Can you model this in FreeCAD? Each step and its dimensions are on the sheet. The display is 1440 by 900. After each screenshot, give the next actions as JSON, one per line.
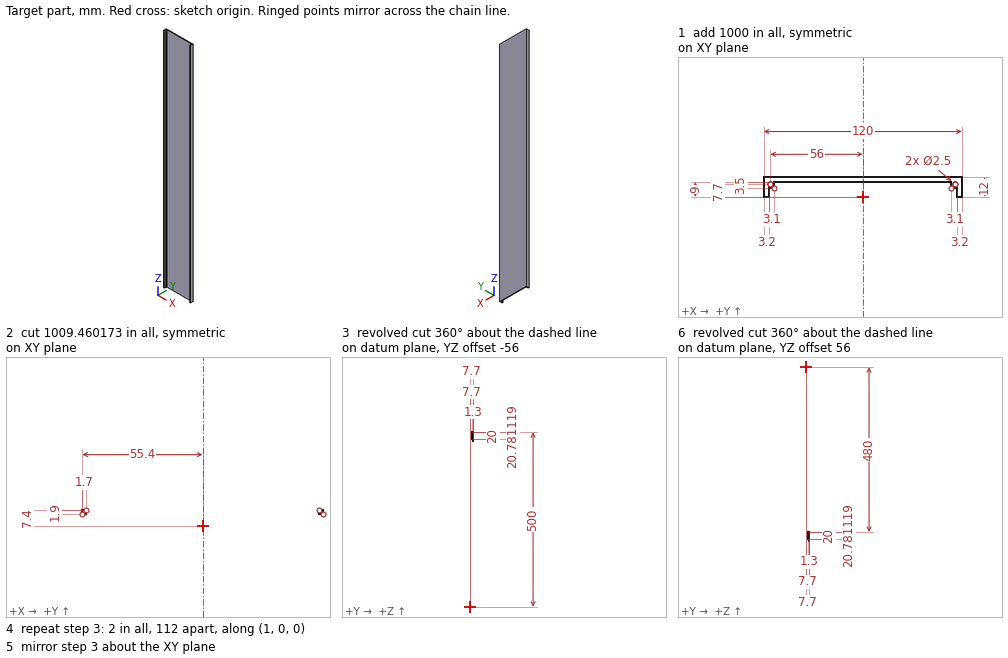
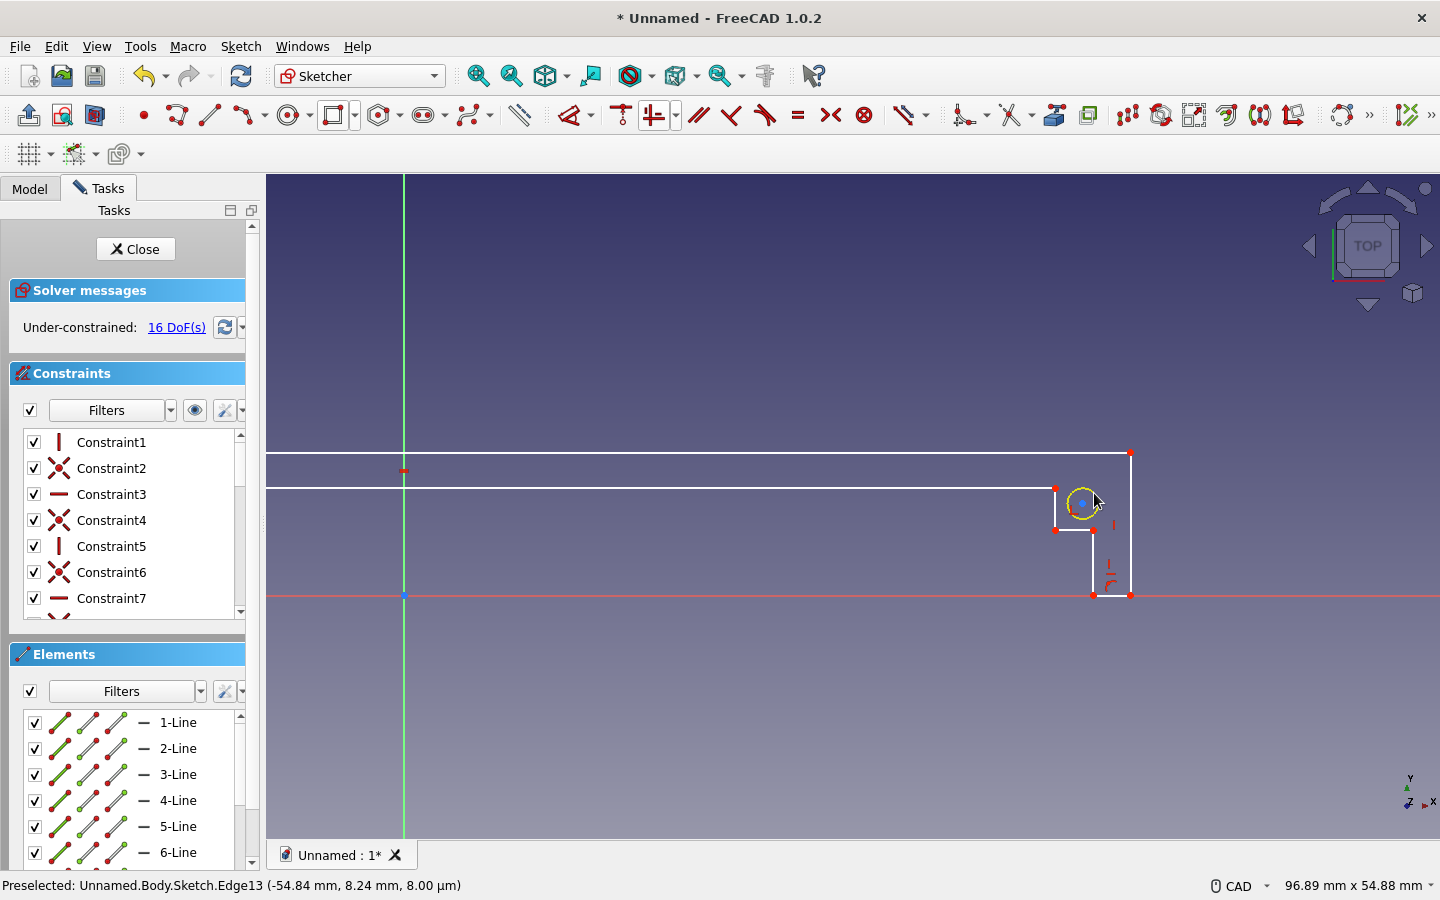
{"action": "left_click", "coordinate": [1094, 493]}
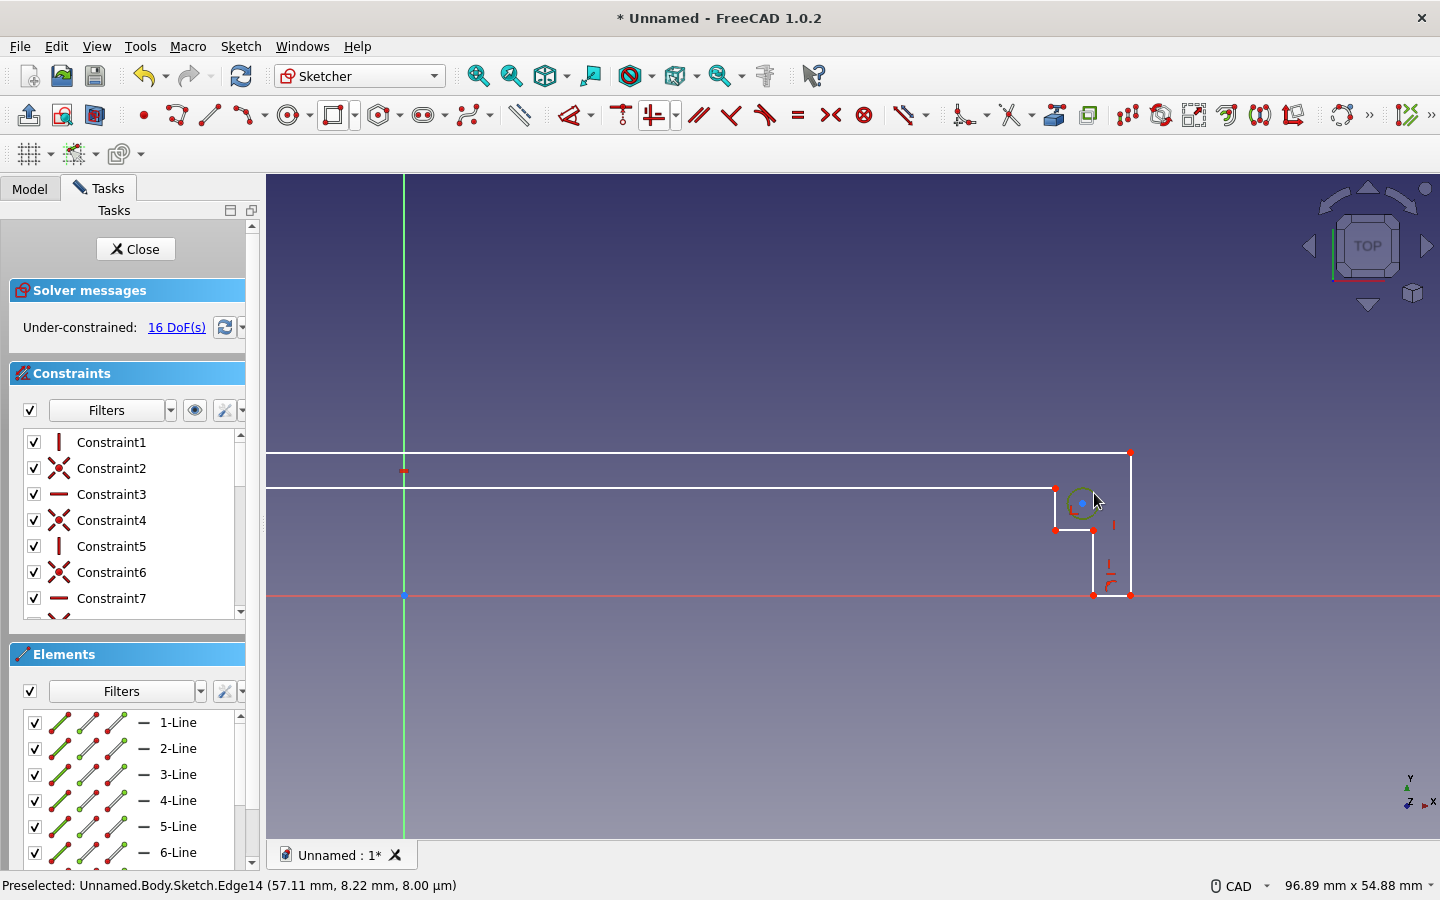
{"action": "key", "text": "e"}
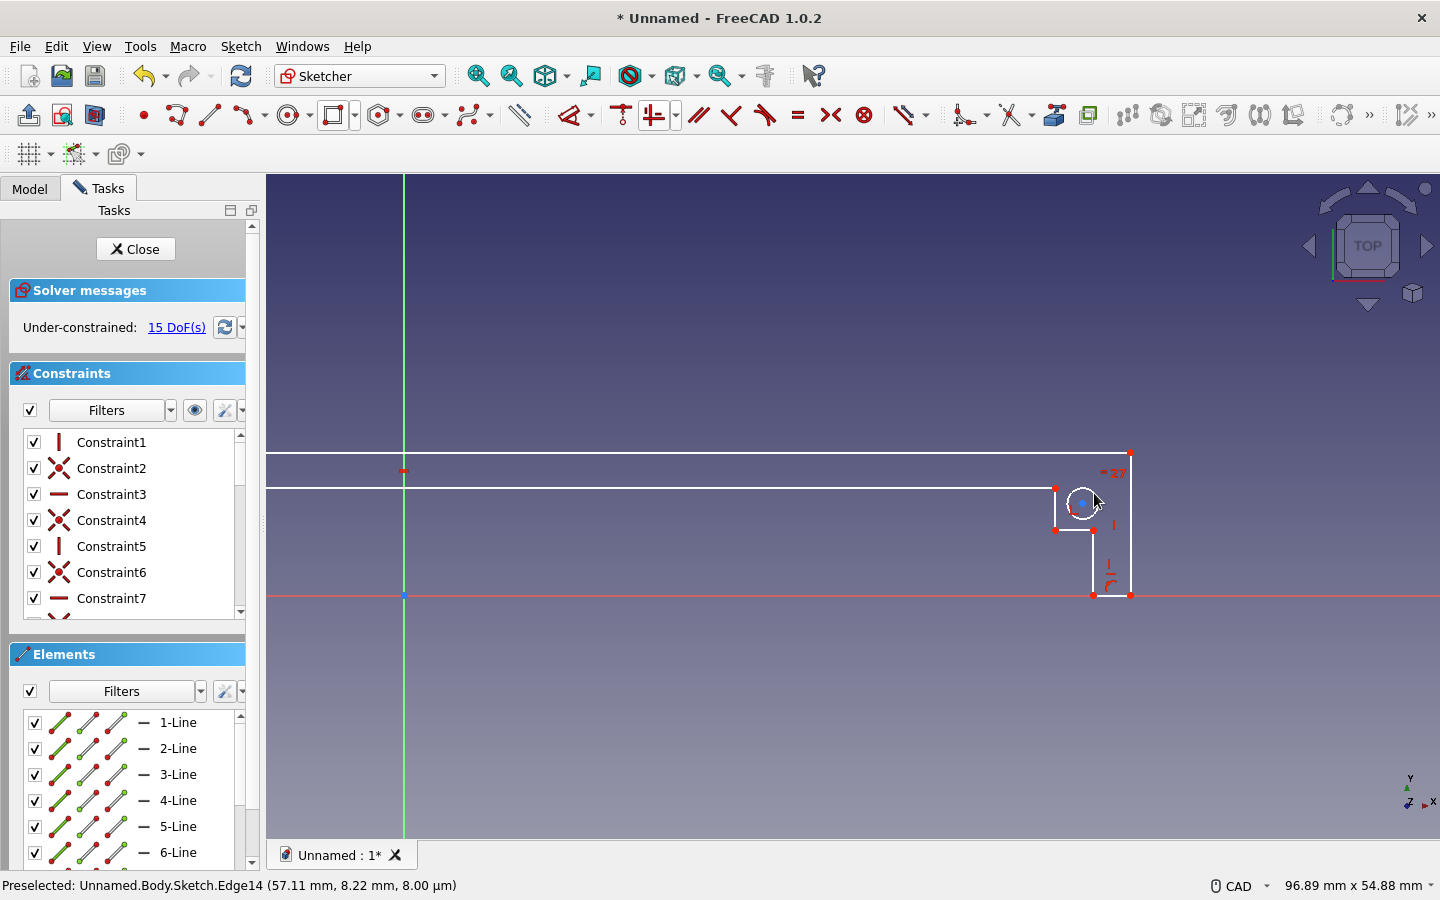
{"action": "scroll", "coordinate": [1095, 493], "scroll_direction": "down", "scroll_amount": 4}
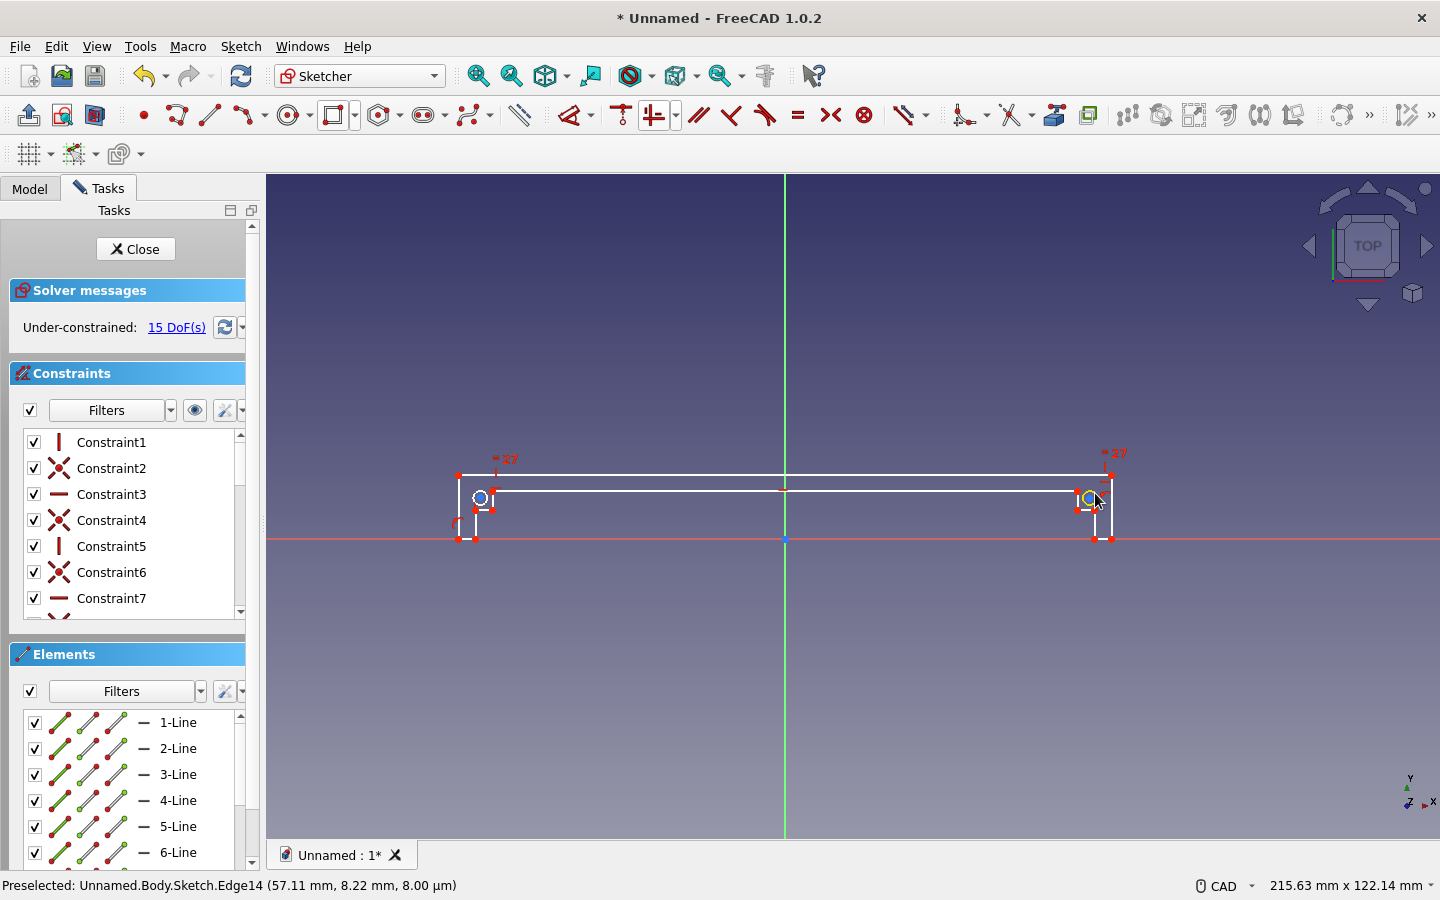
{"action": "left_click", "coordinate": [480, 498]}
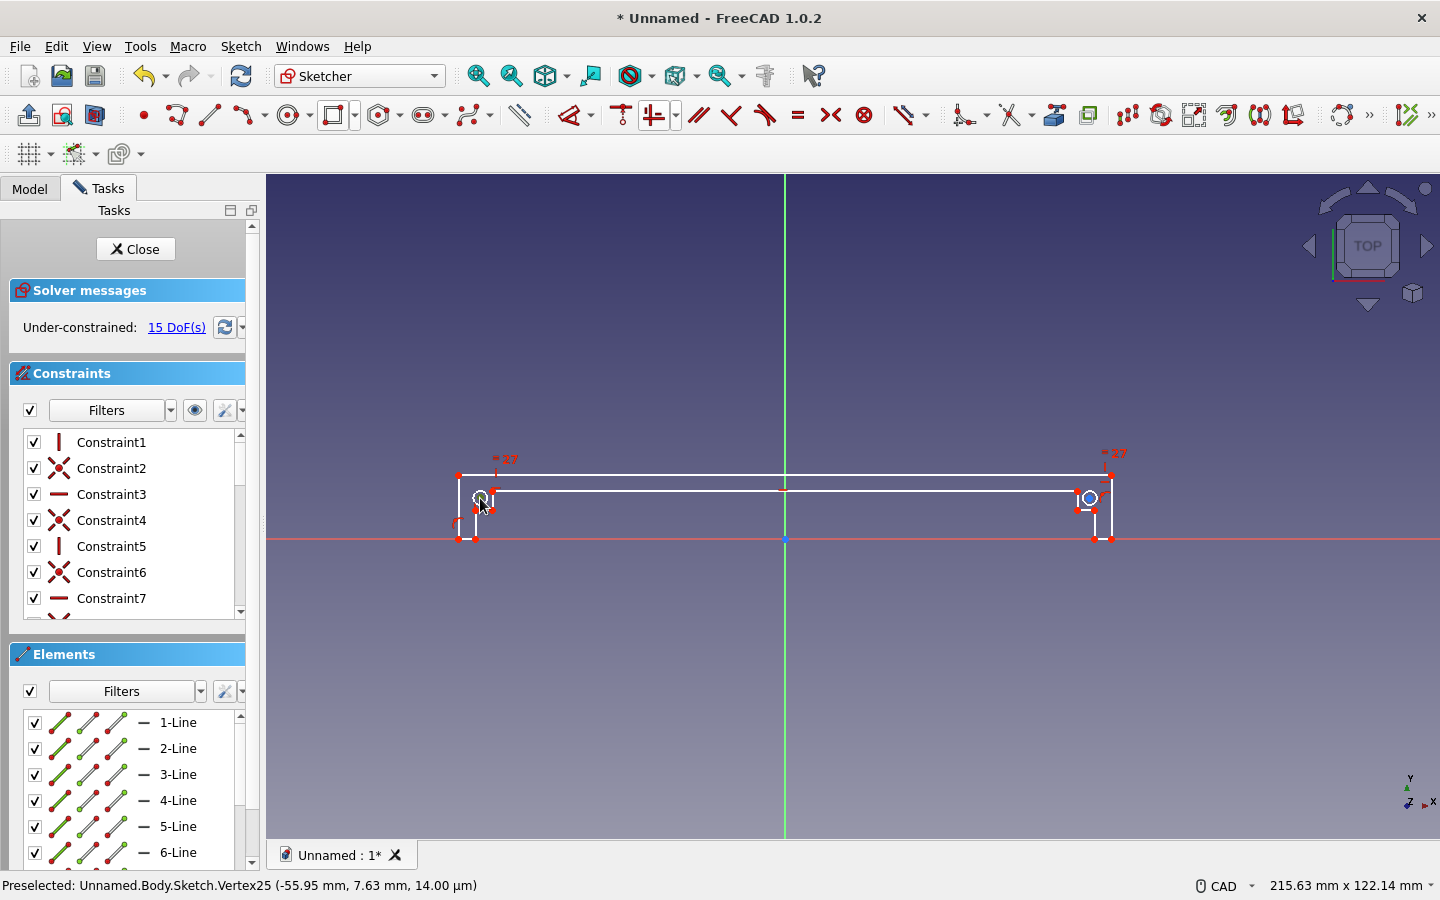
{"action": "left_click", "coordinate": [1090, 498]}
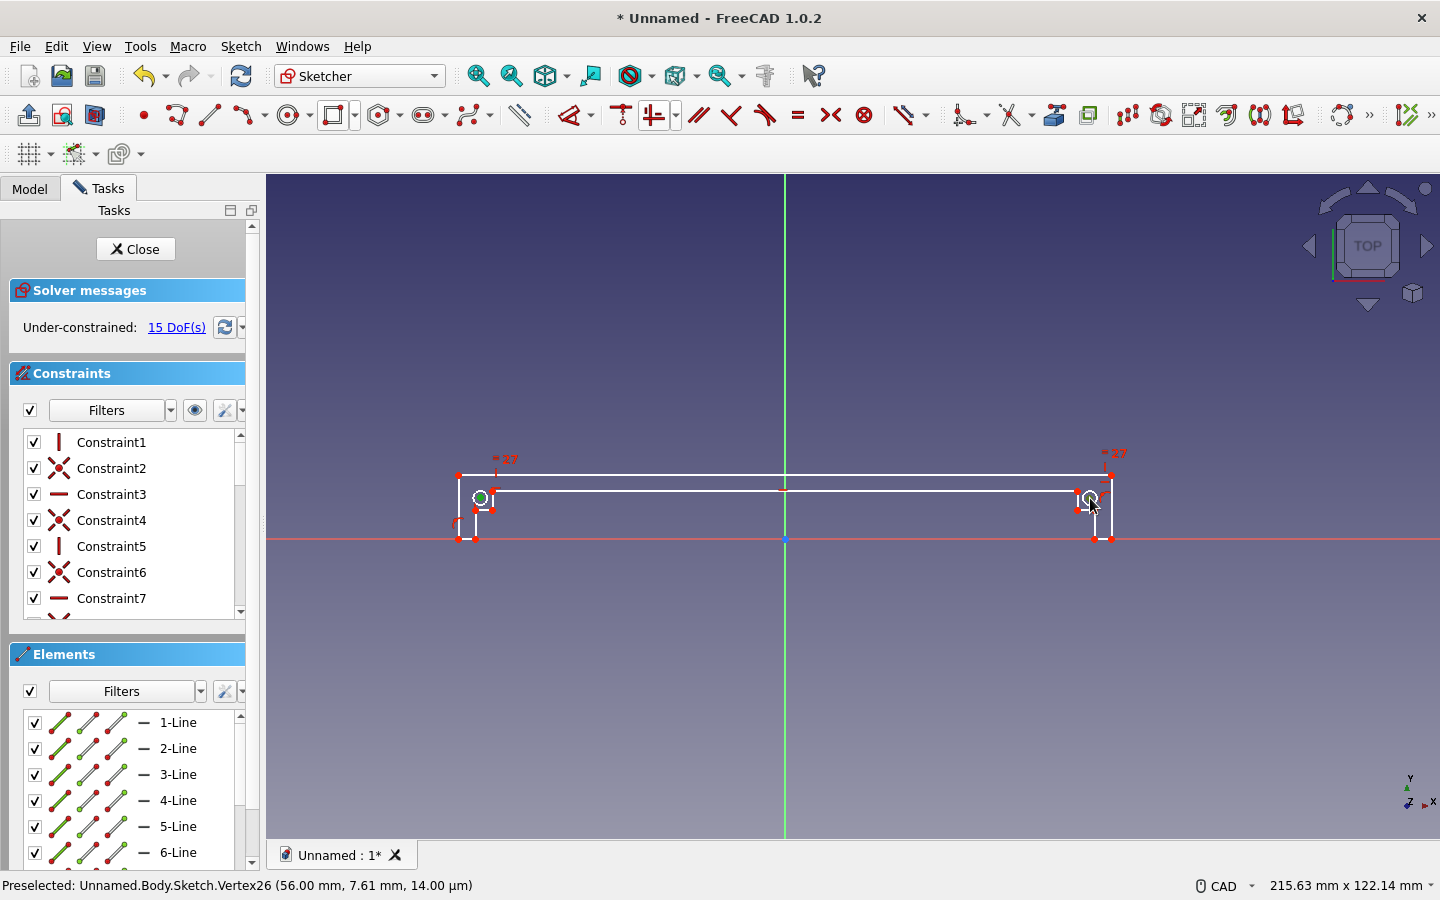
{"action": "left_click", "coordinate": [785, 768]}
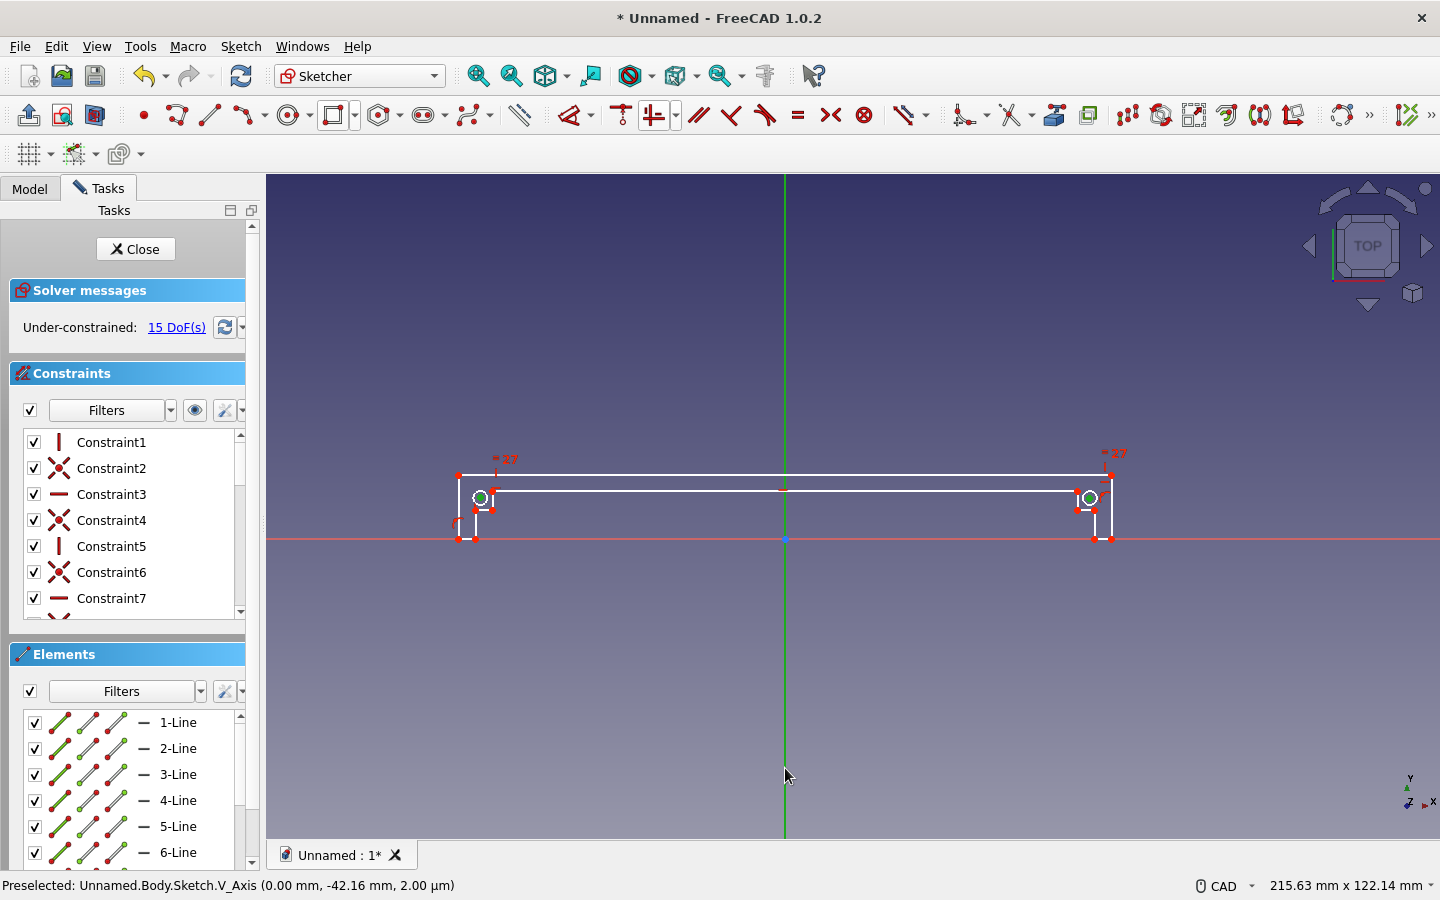
{"action": "key", "text": "s"}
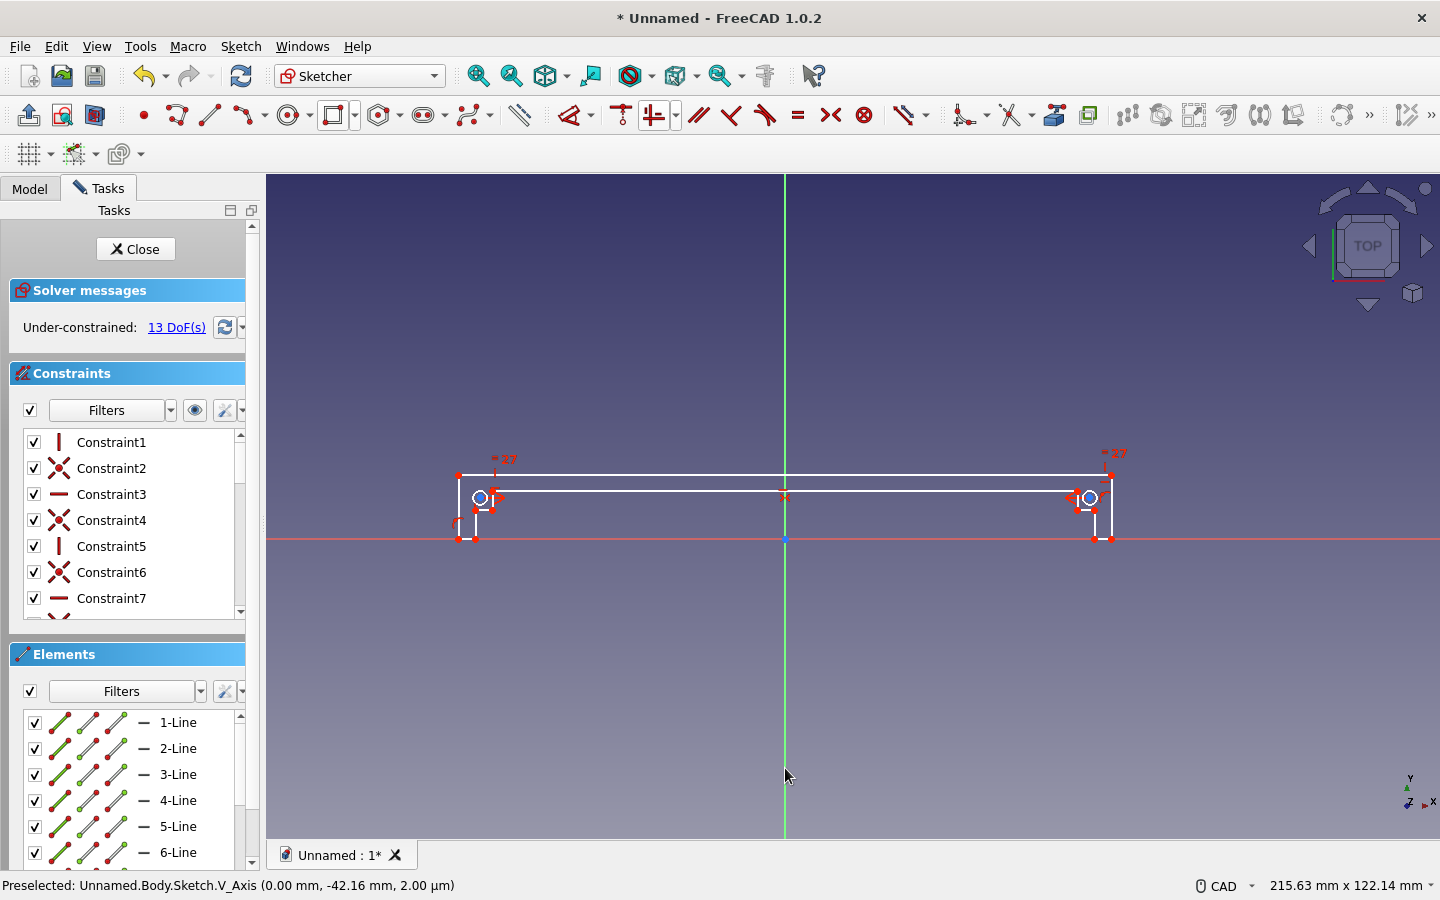
{"action": "left_click", "coordinate": [493, 510]}